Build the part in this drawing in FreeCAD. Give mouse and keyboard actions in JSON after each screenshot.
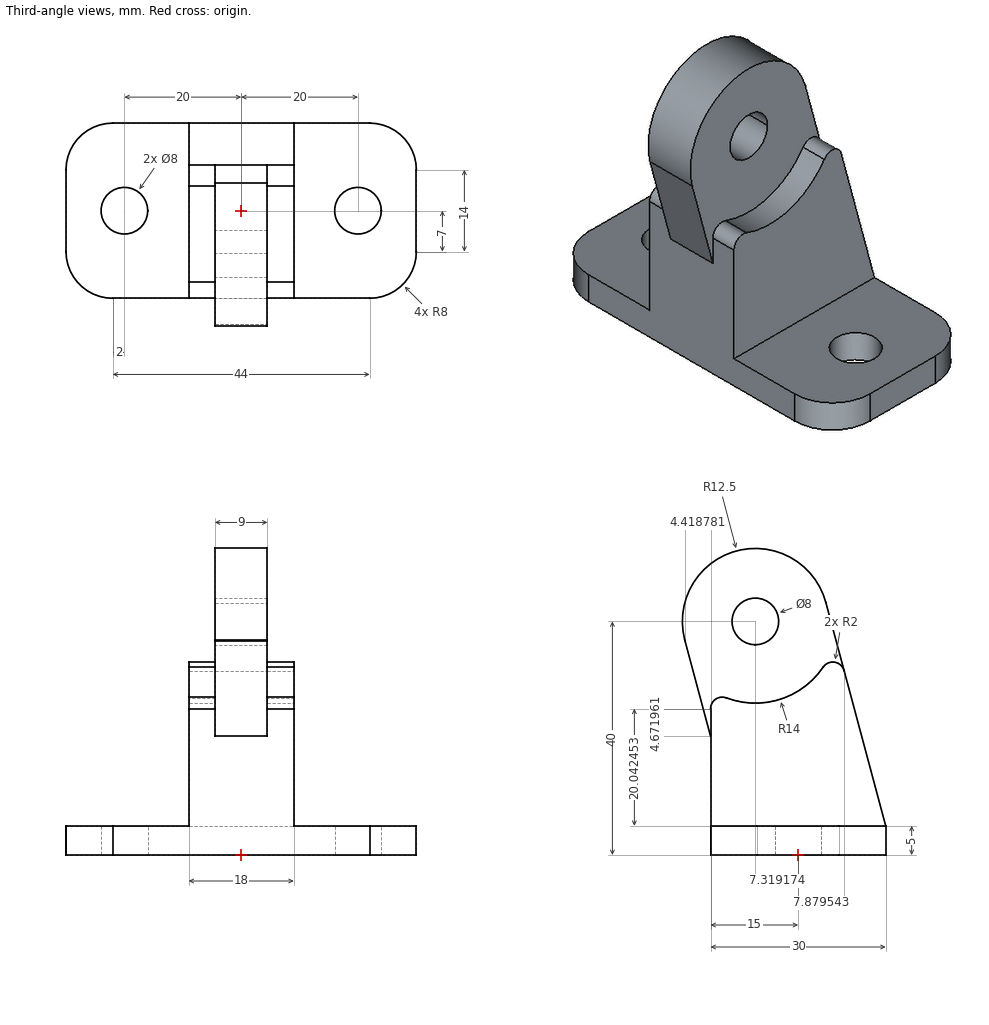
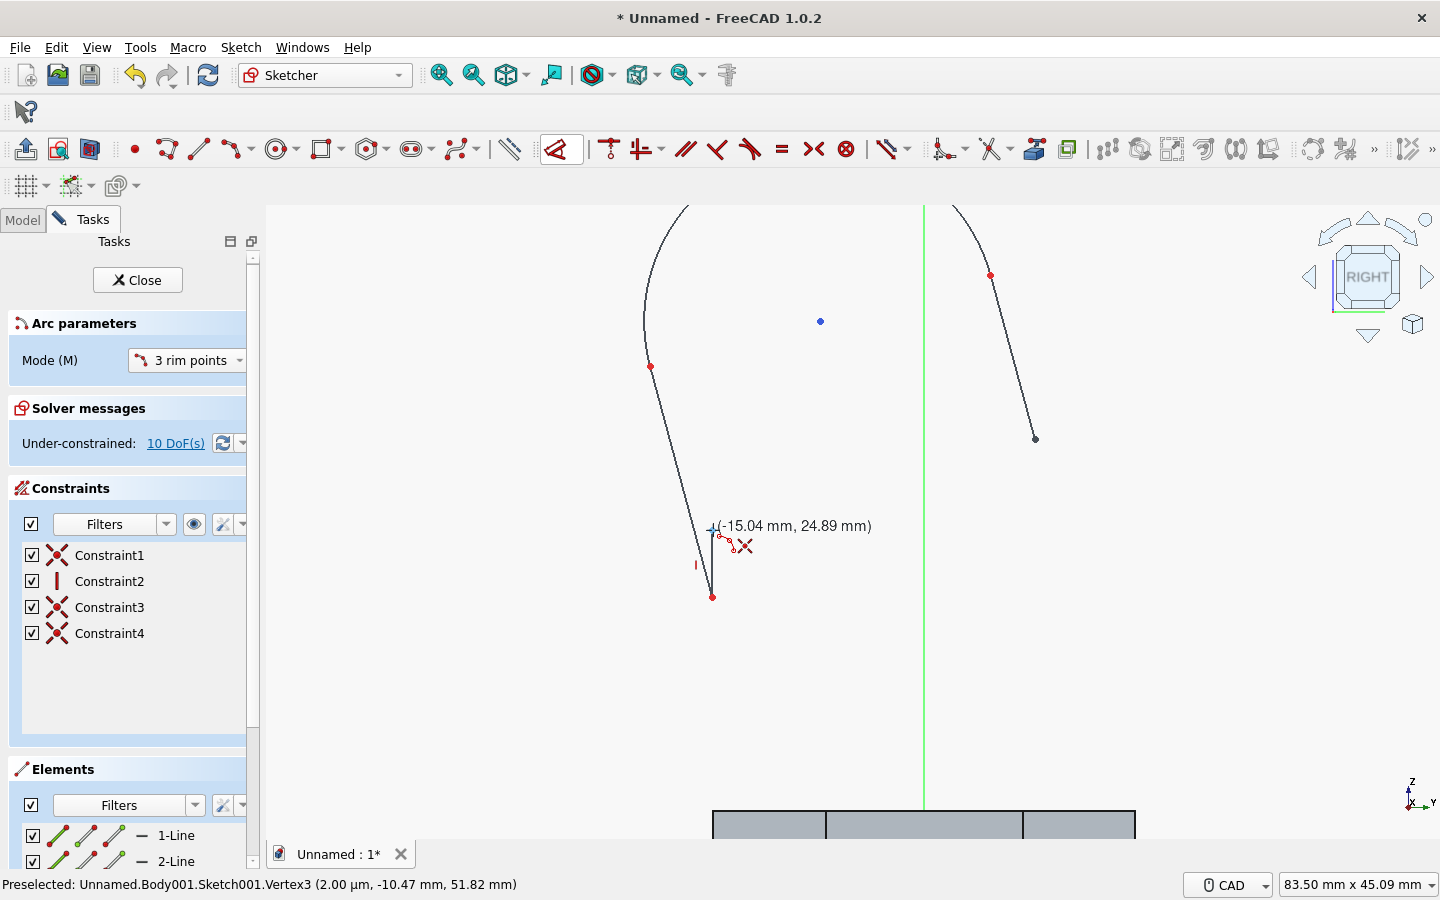
{"action": "left_click", "coordinate": [712, 530]}
{"action": "left_click", "coordinate": [751, 503]}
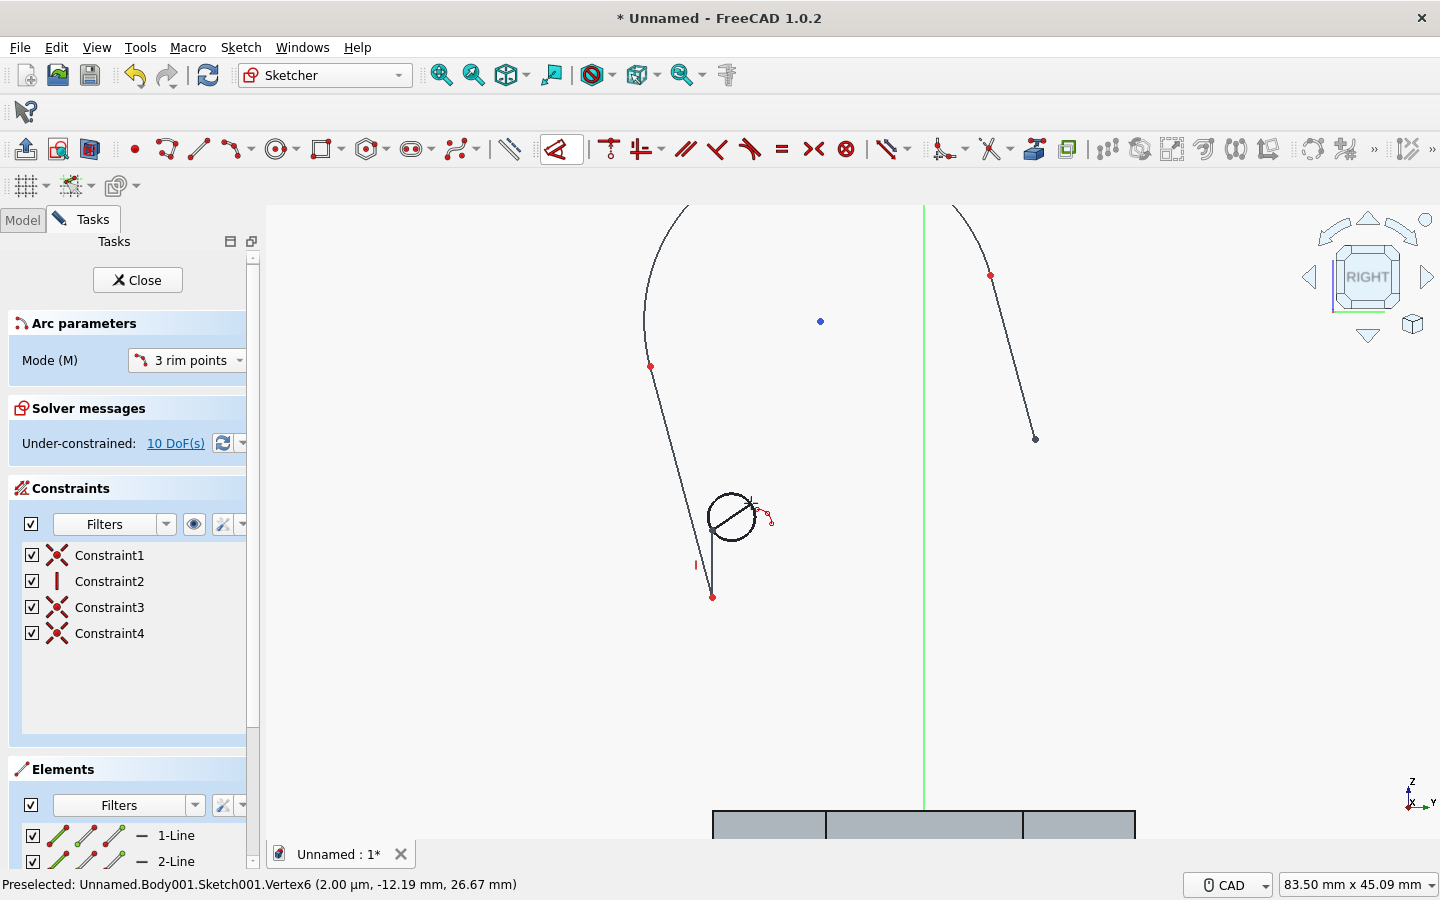
{"action": "scroll", "coordinate": [725, 506], "scroll_direction": "up", "scroll_amount": 2}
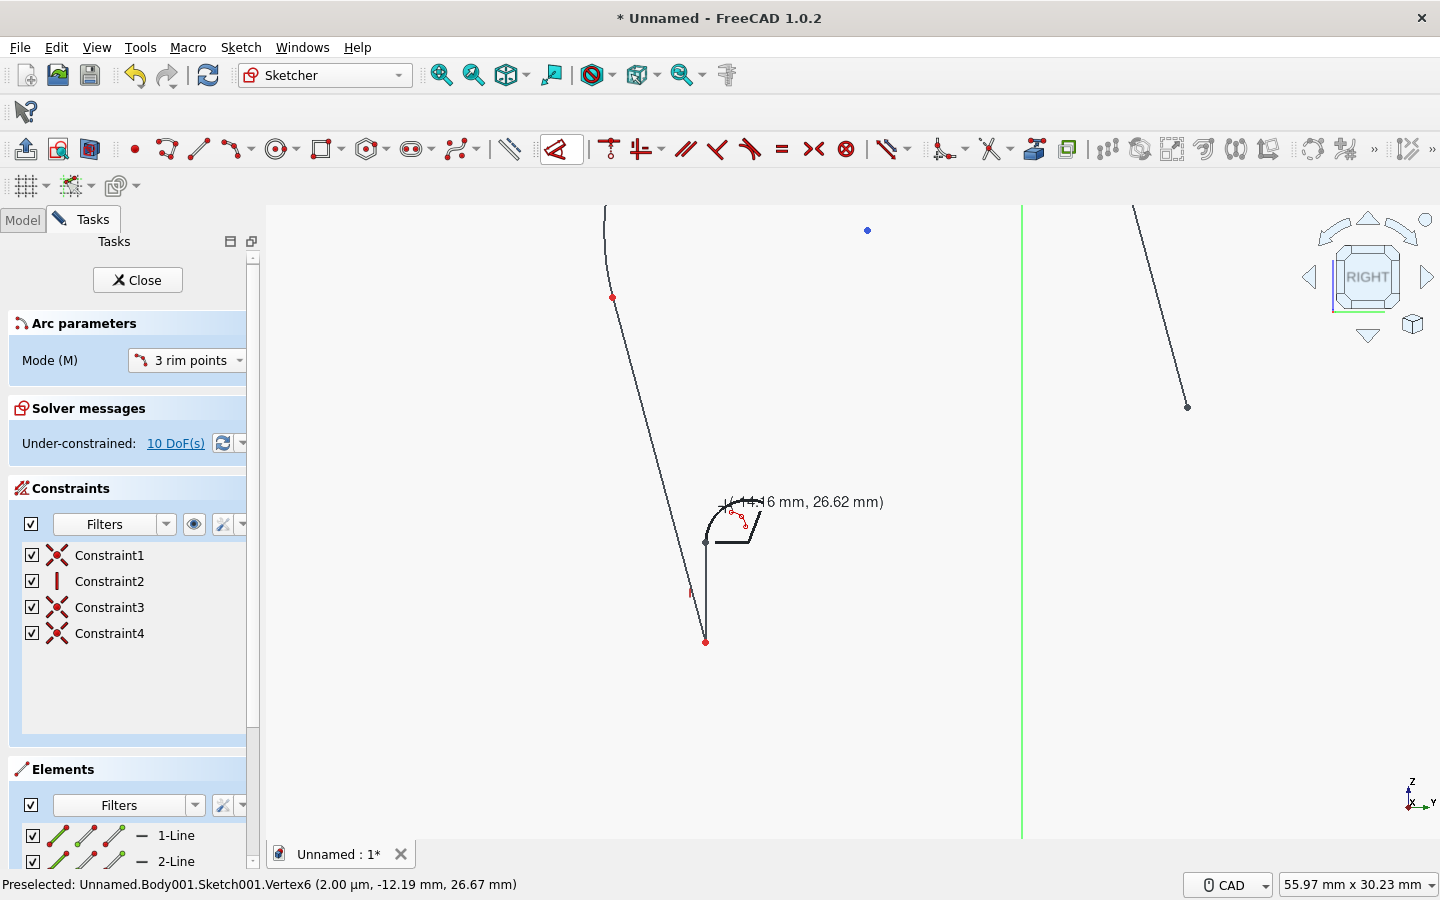
{"action": "left_click", "coordinate": [725, 506]}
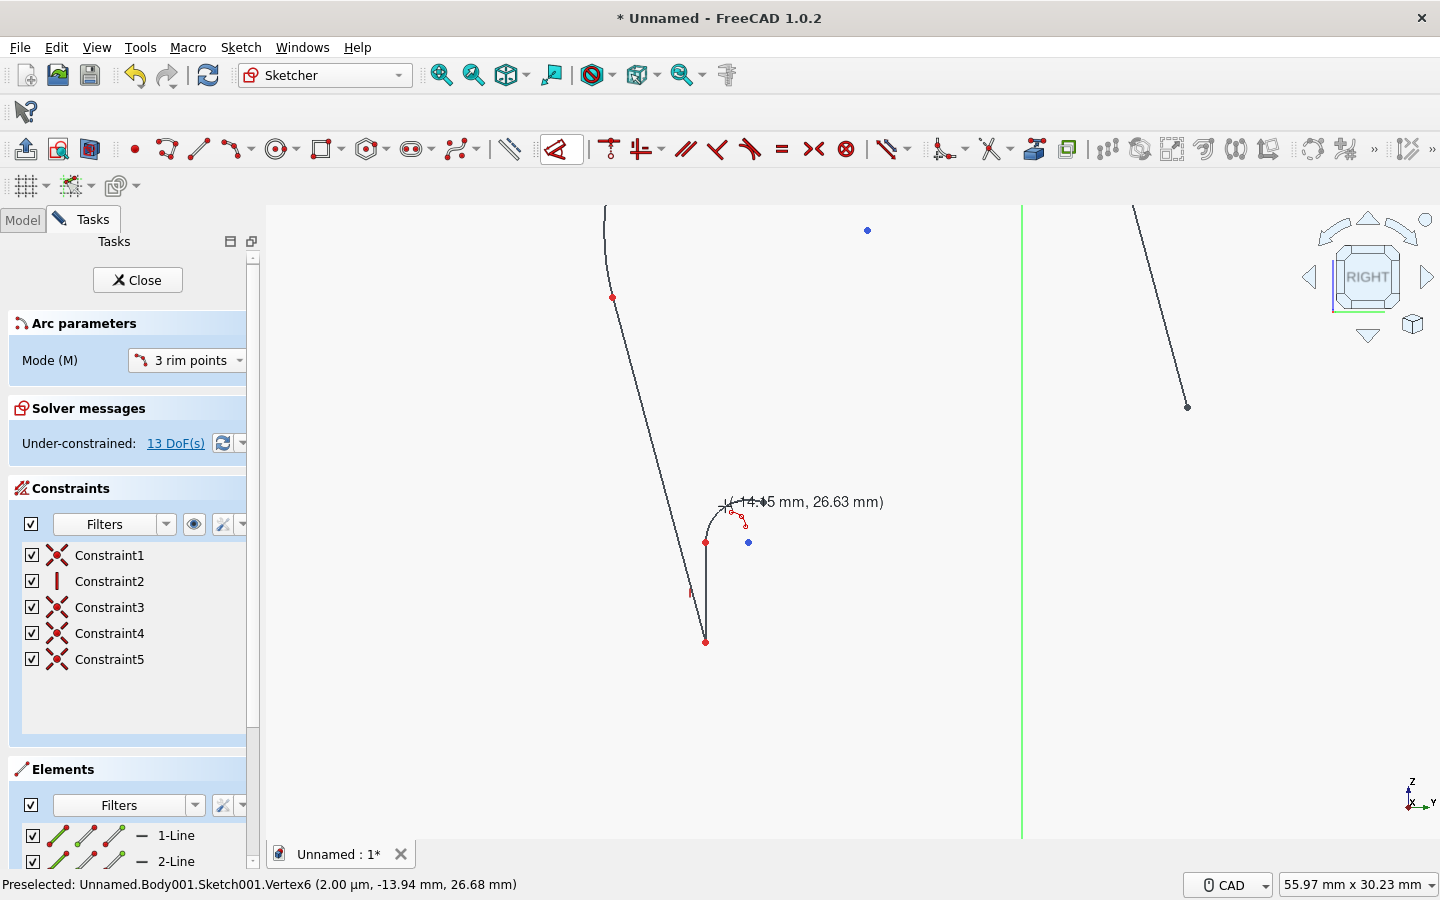
{"action": "left_click", "coordinate": [764, 503]}
{"action": "left_click", "coordinate": [1112, 391]}
{"action": "left_click", "coordinate": [957, 507]}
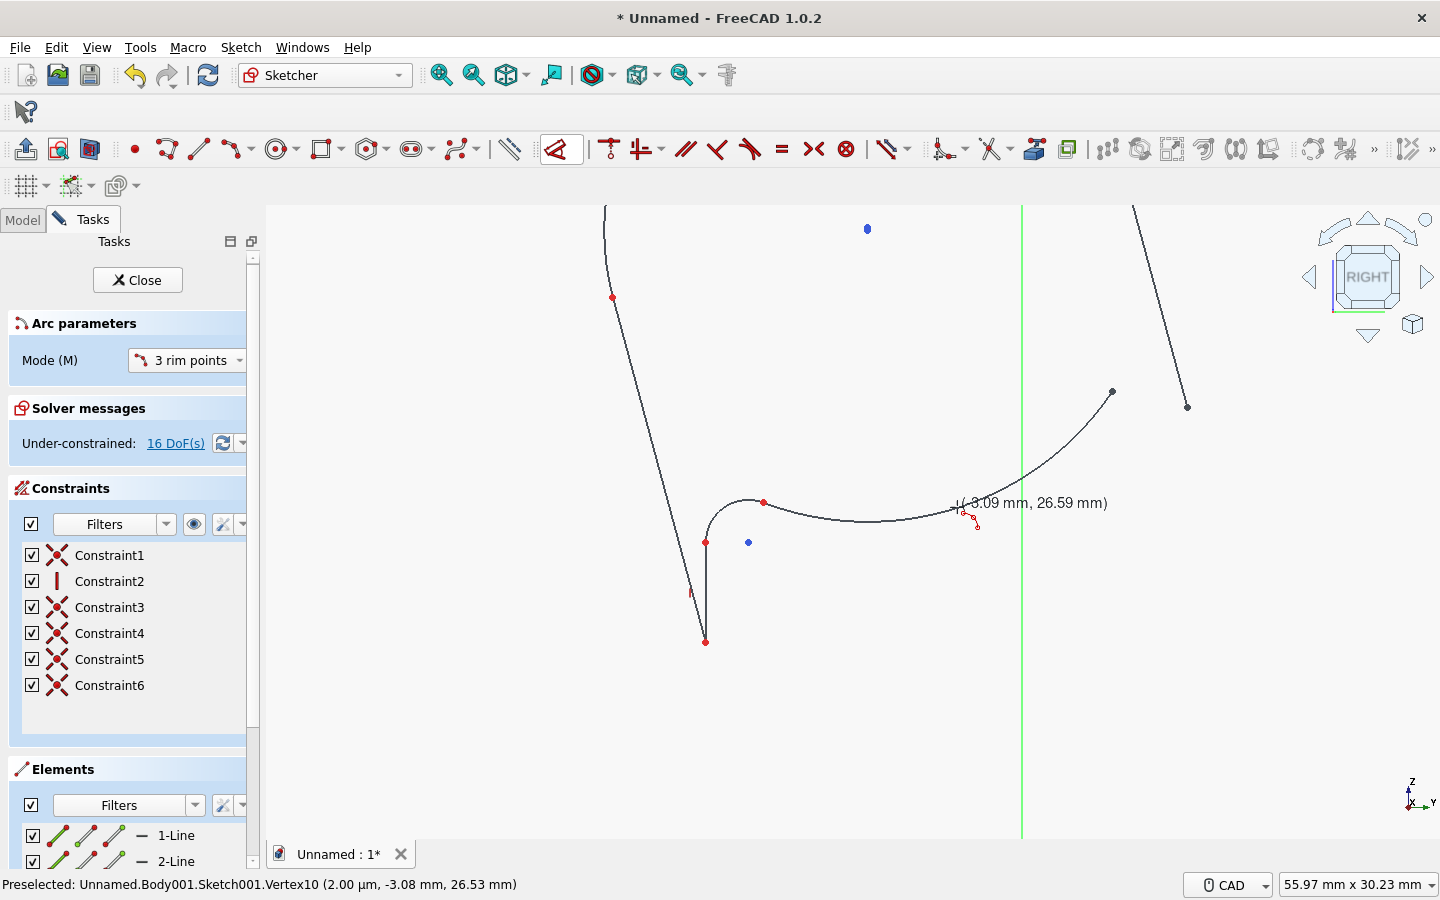
{"action": "left_click", "coordinate": [1112, 392]}
{"action": "left_click", "coordinate": [1187, 407]}
{"action": "left_click", "coordinate": [1154, 373]}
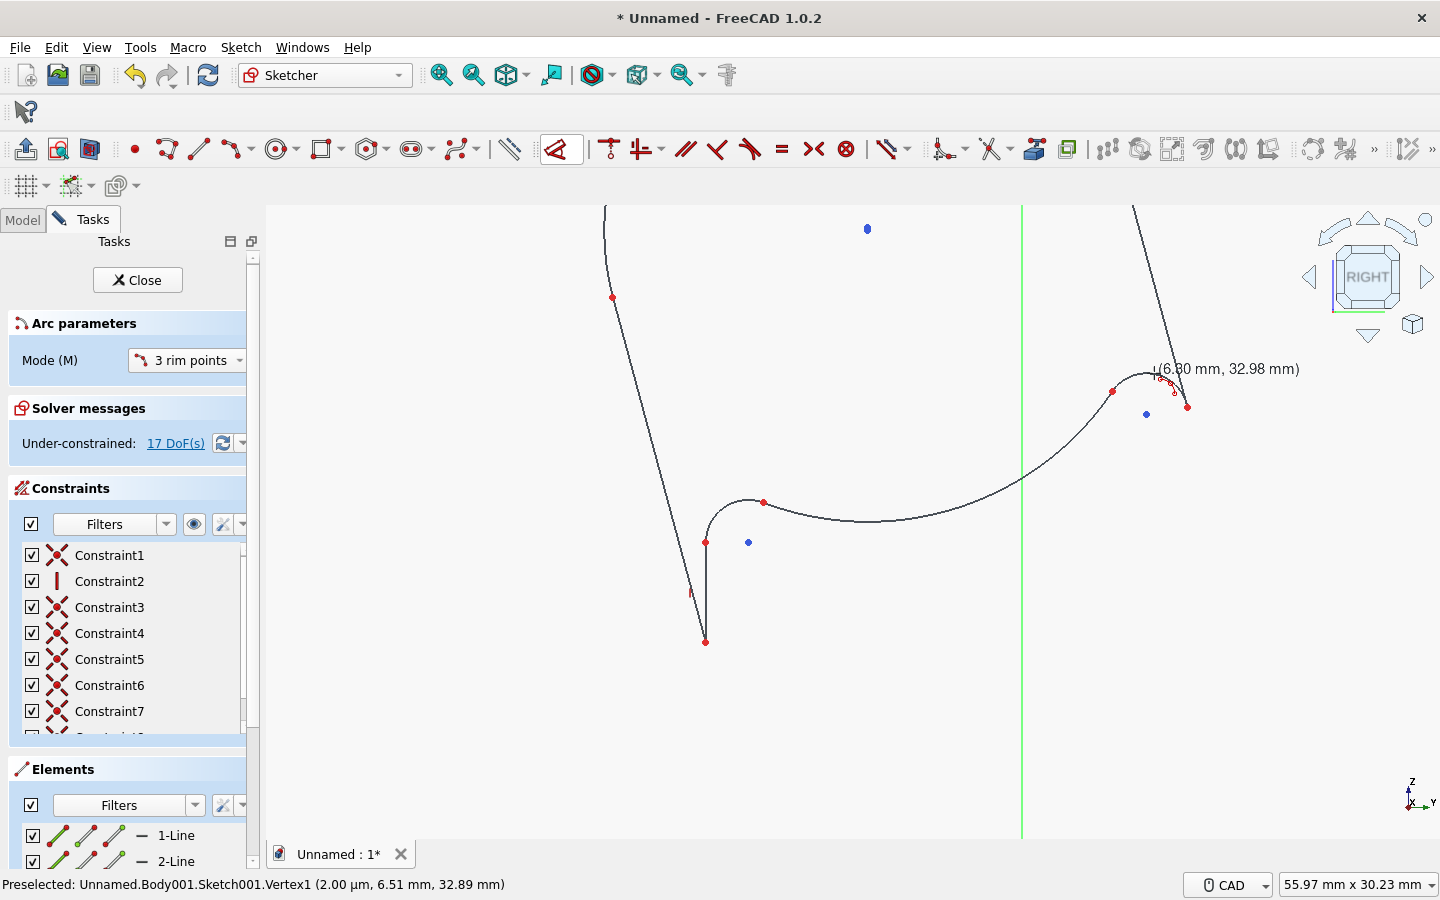
{"action": "left_click", "coordinate": [276, 150]}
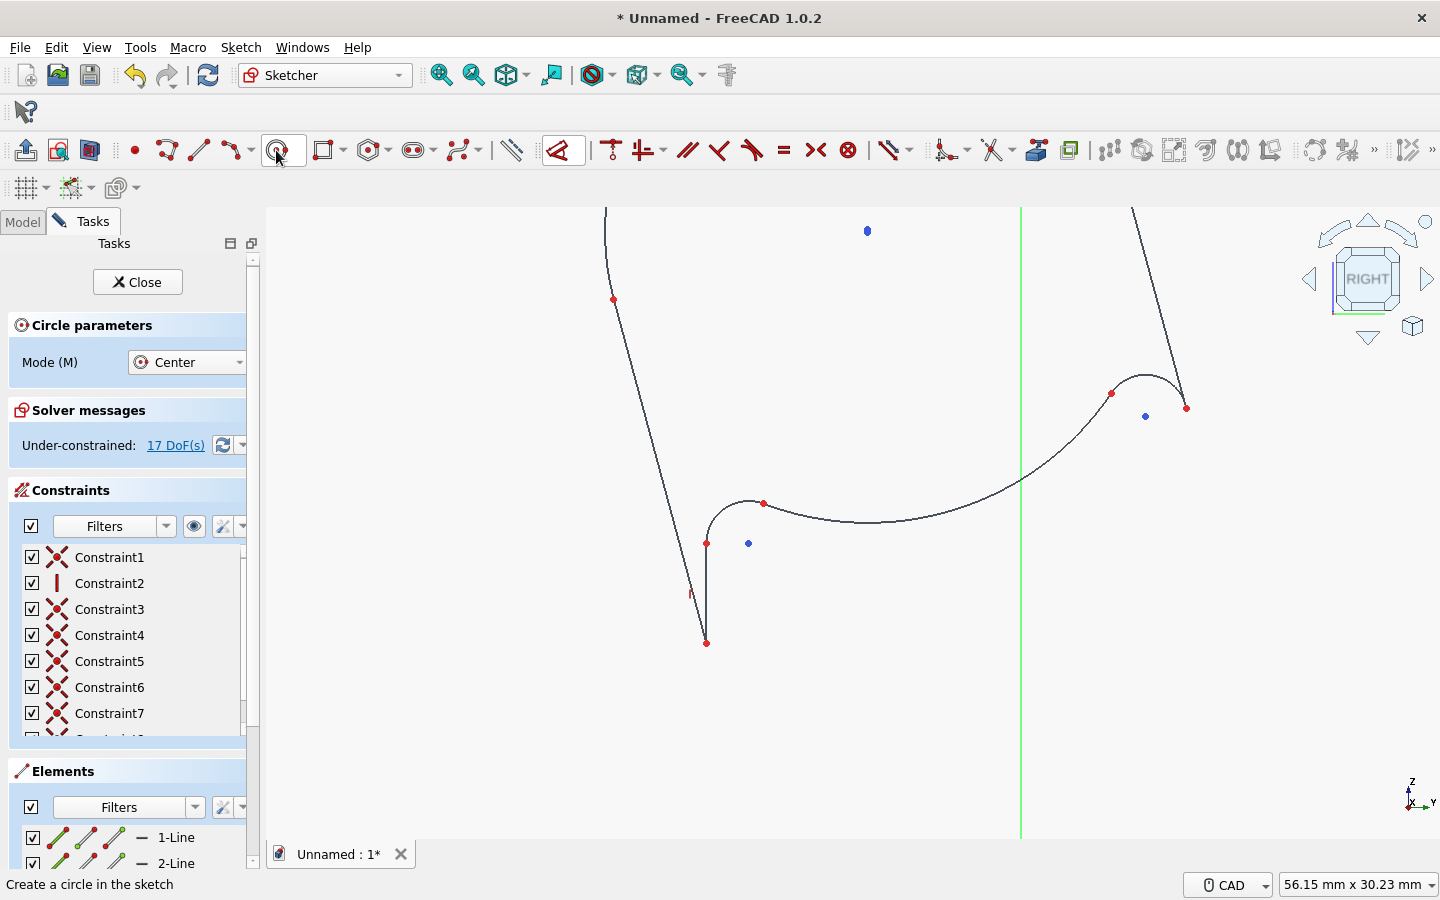
{"action": "scroll", "coordinate": [717, 525], "scroll_direction": "down", "scroll_amount": 5}